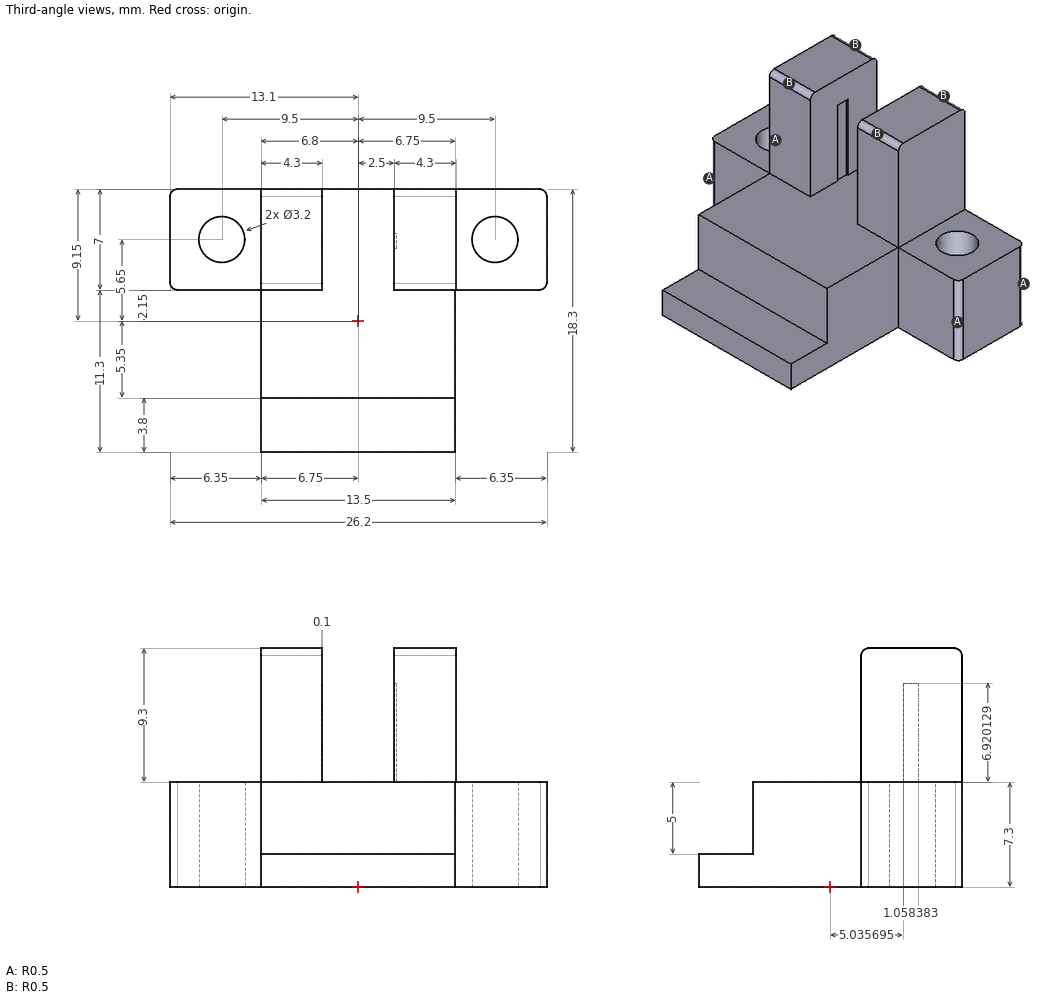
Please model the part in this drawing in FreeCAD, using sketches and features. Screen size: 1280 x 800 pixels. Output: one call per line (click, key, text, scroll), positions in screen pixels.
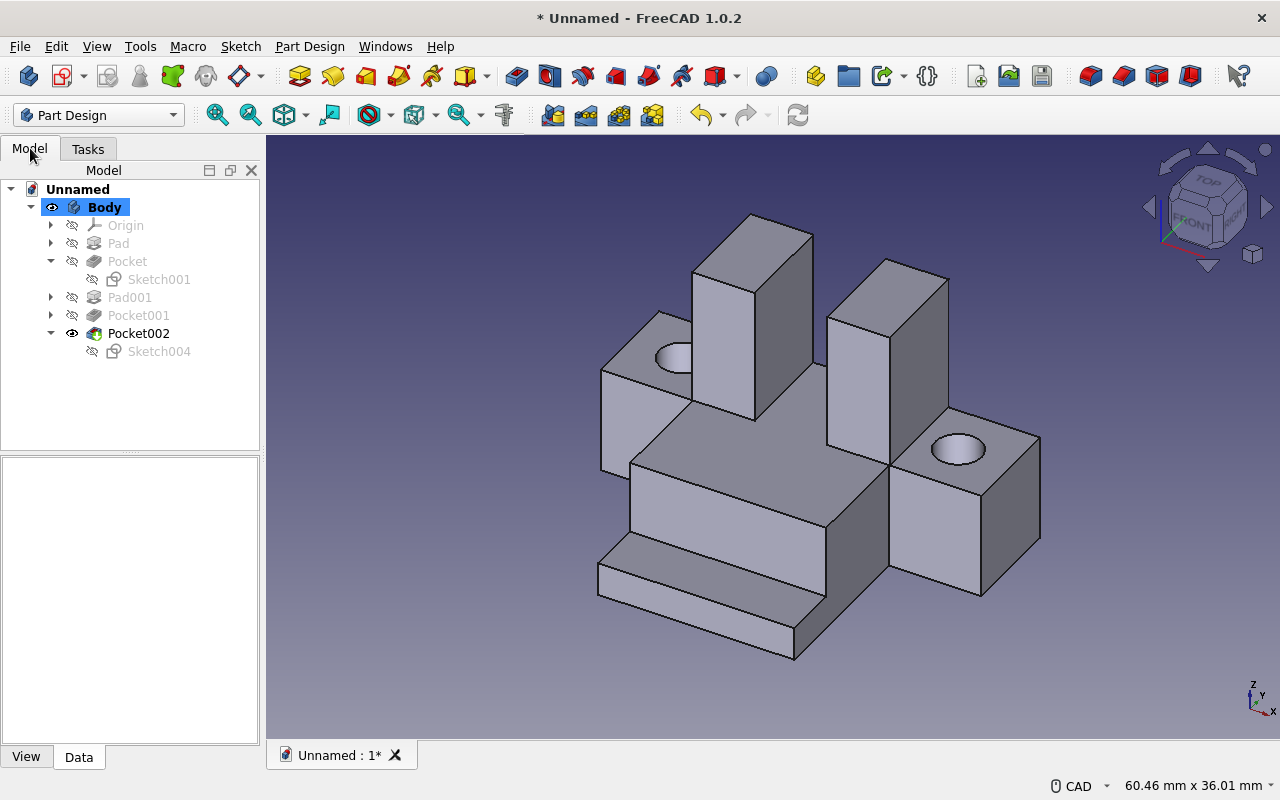
click(51, 225)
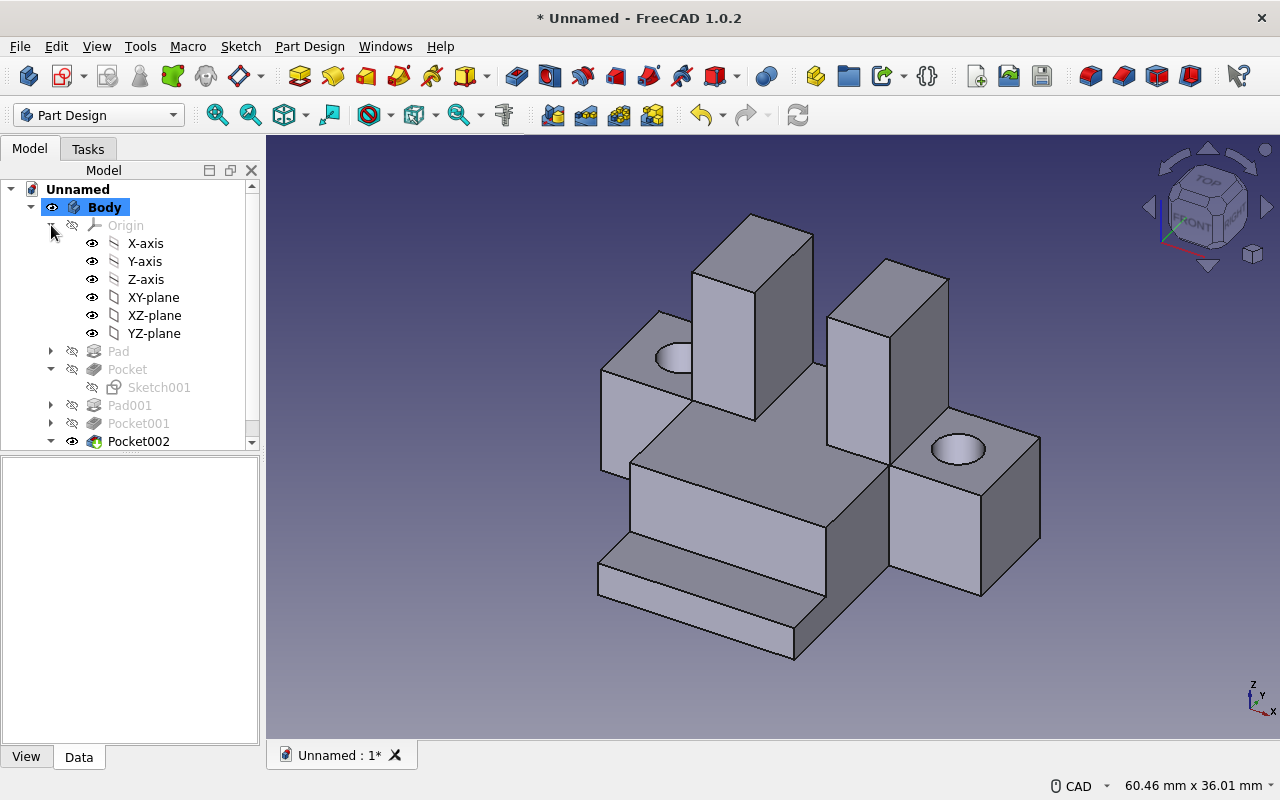
click(137, 333)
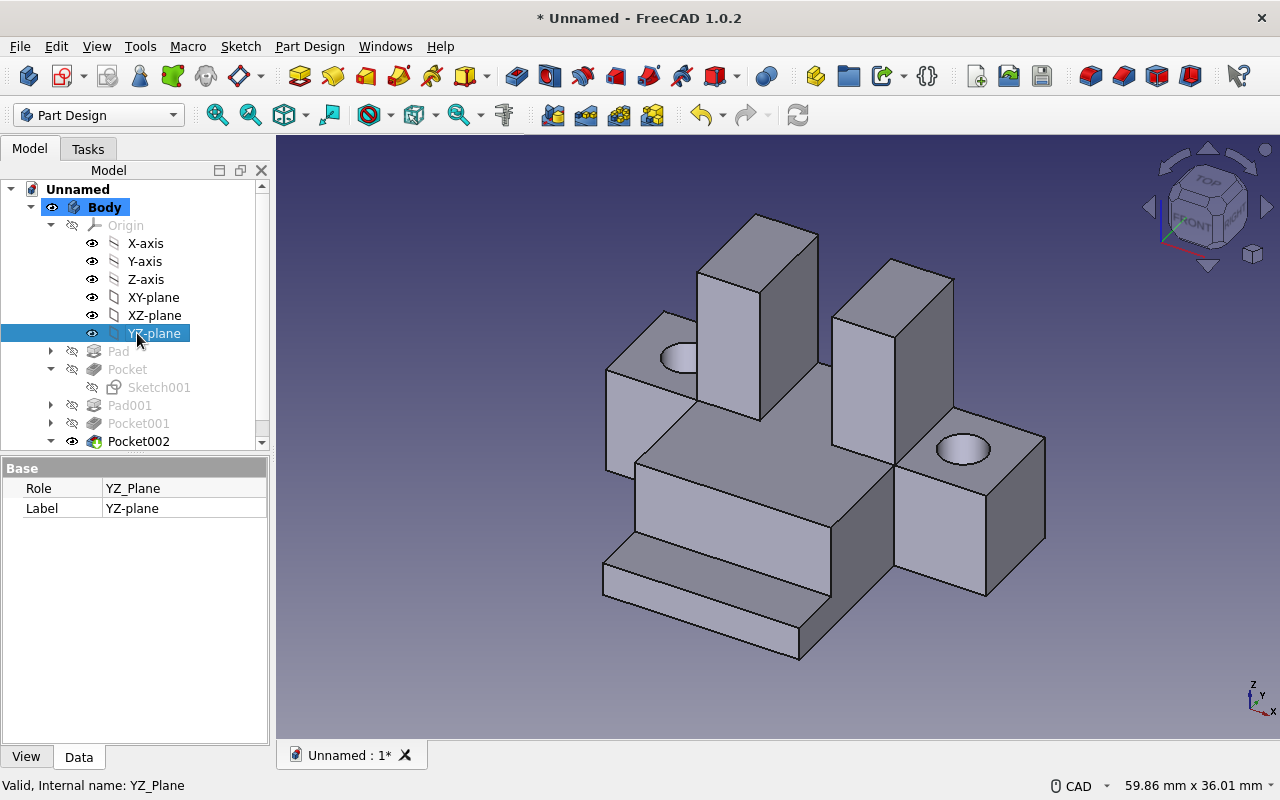
click(238, 76)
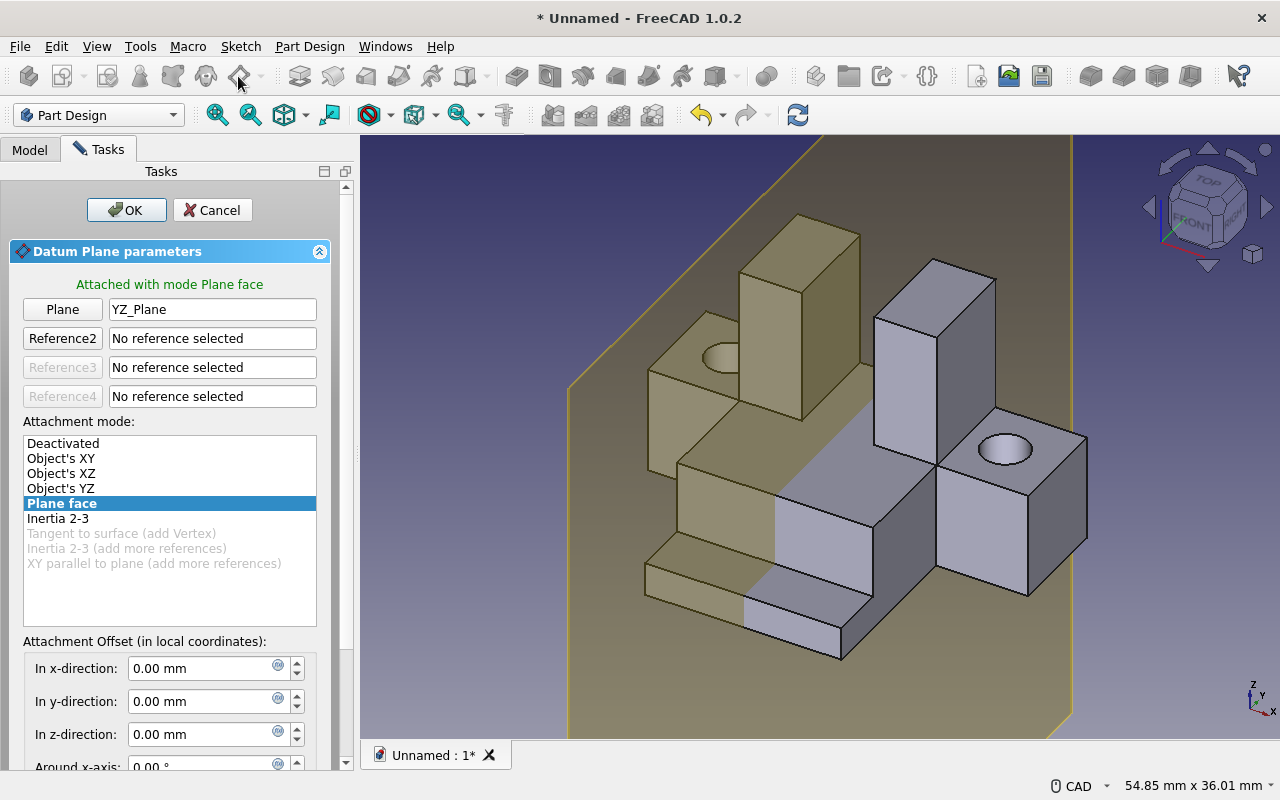
triple_click(210, 734)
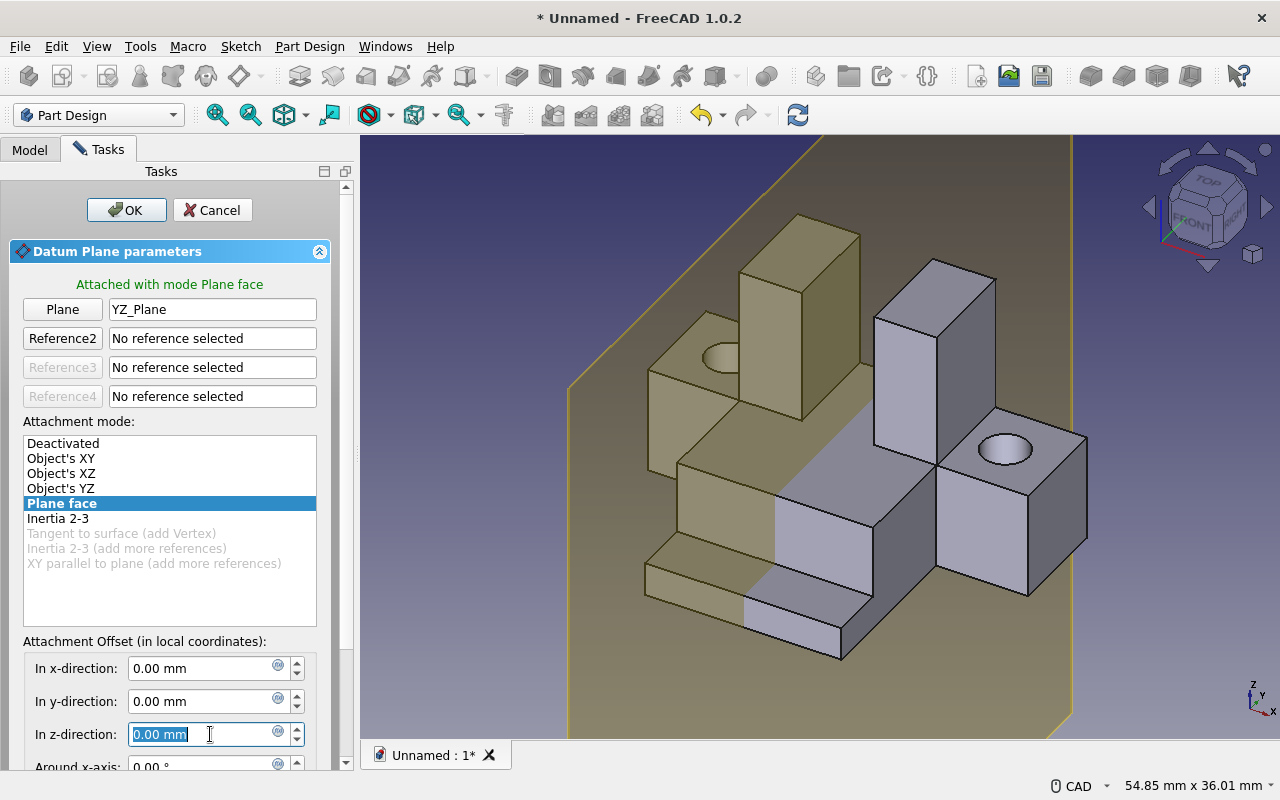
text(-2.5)
key(Tab)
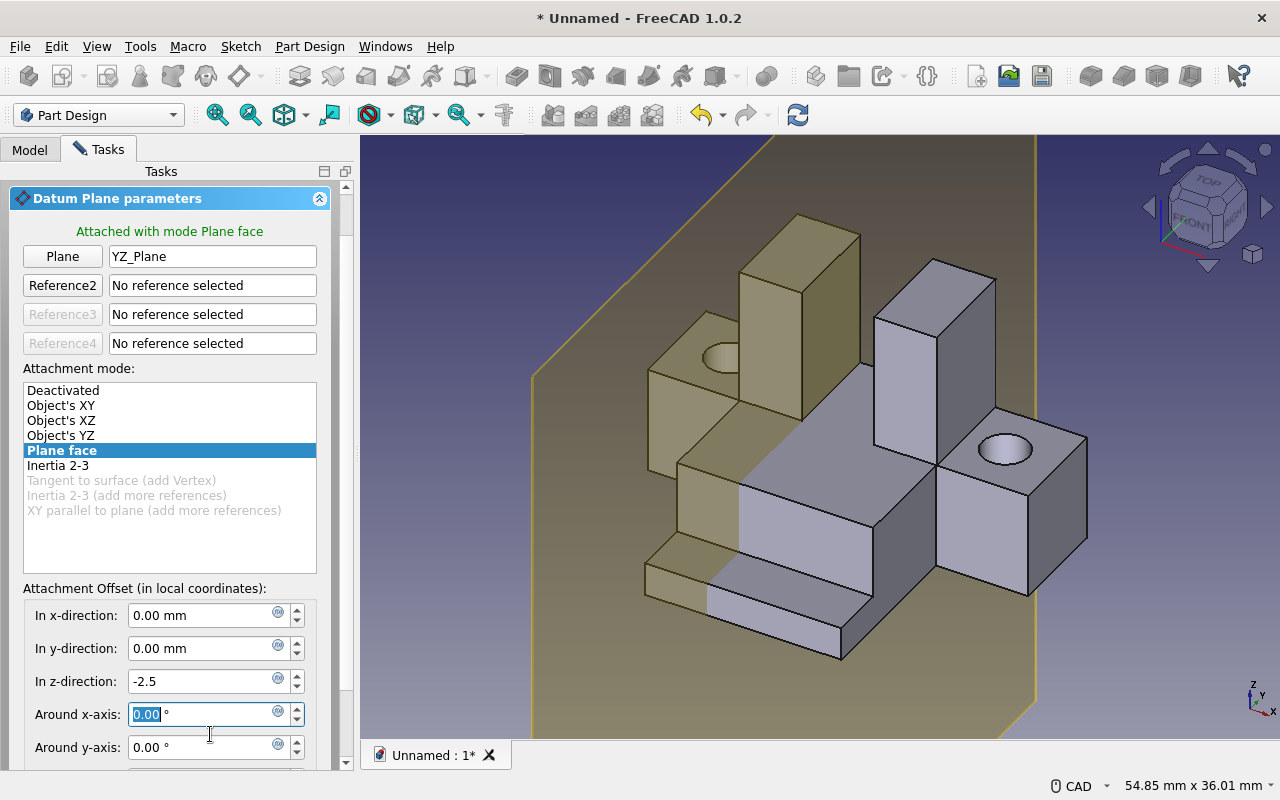
scroll(346, 476, up, 2)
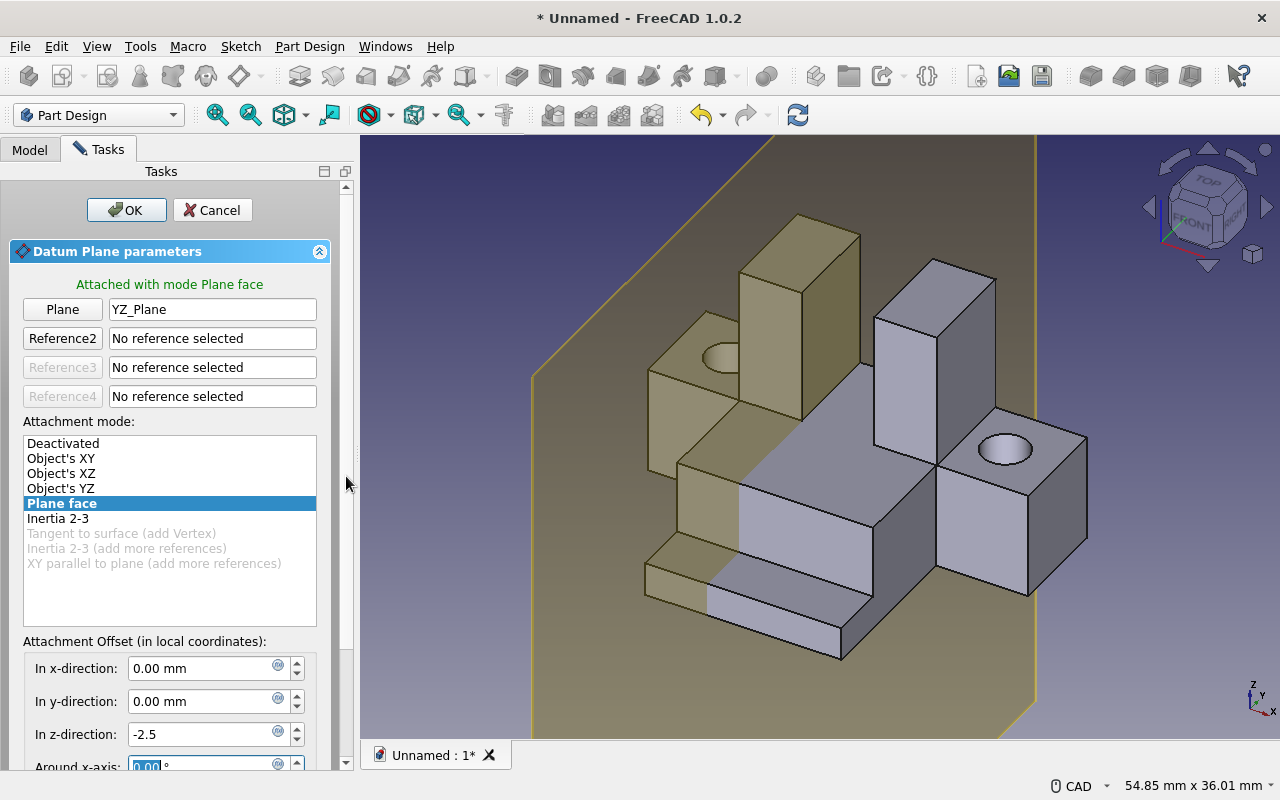
click(127, 210)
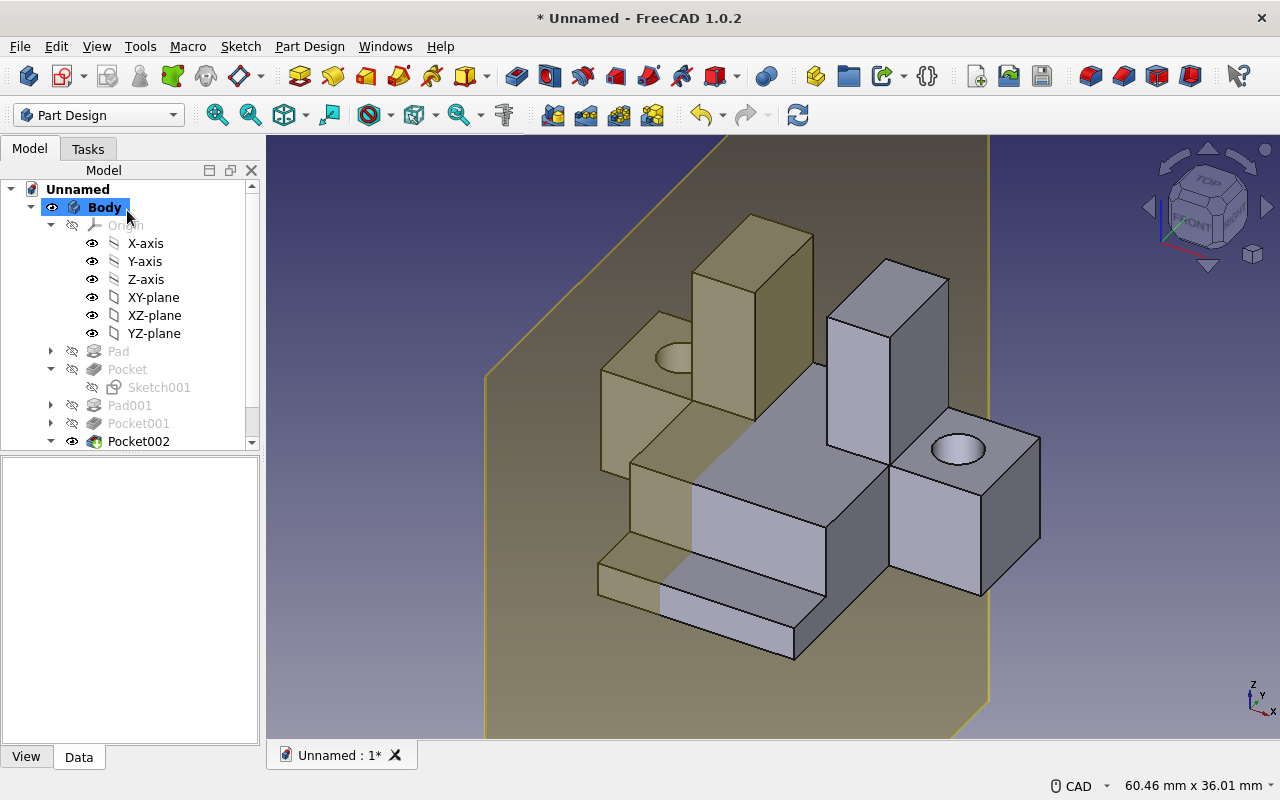
scroll(101, 311, down, 3)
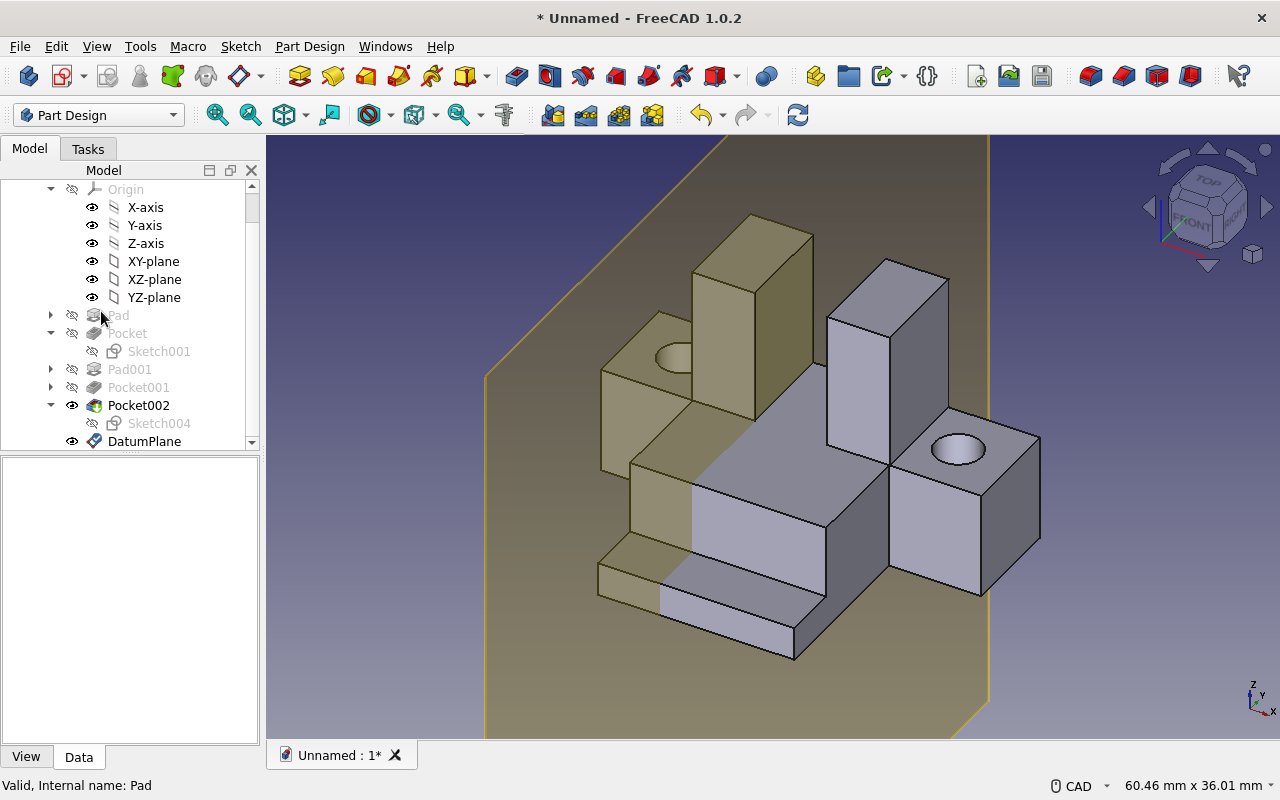
click(117, 441)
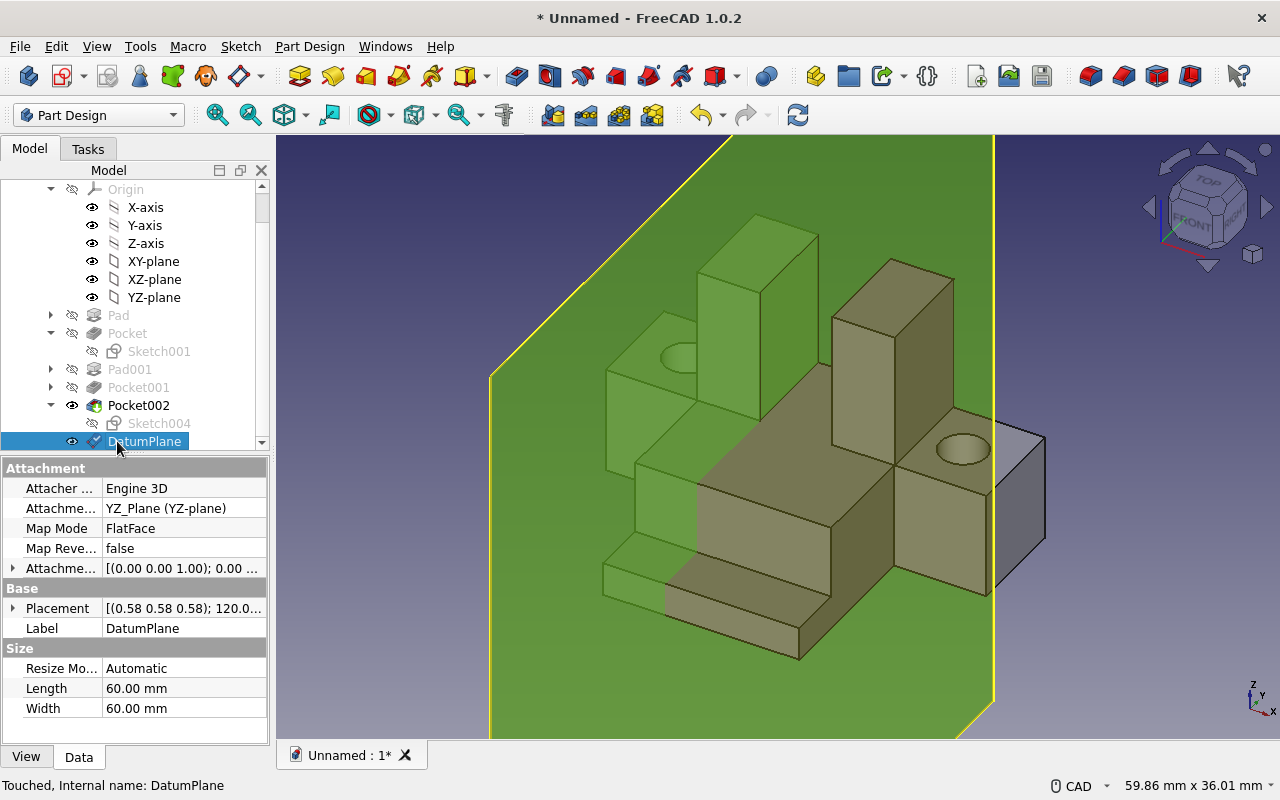
click(62, 76)